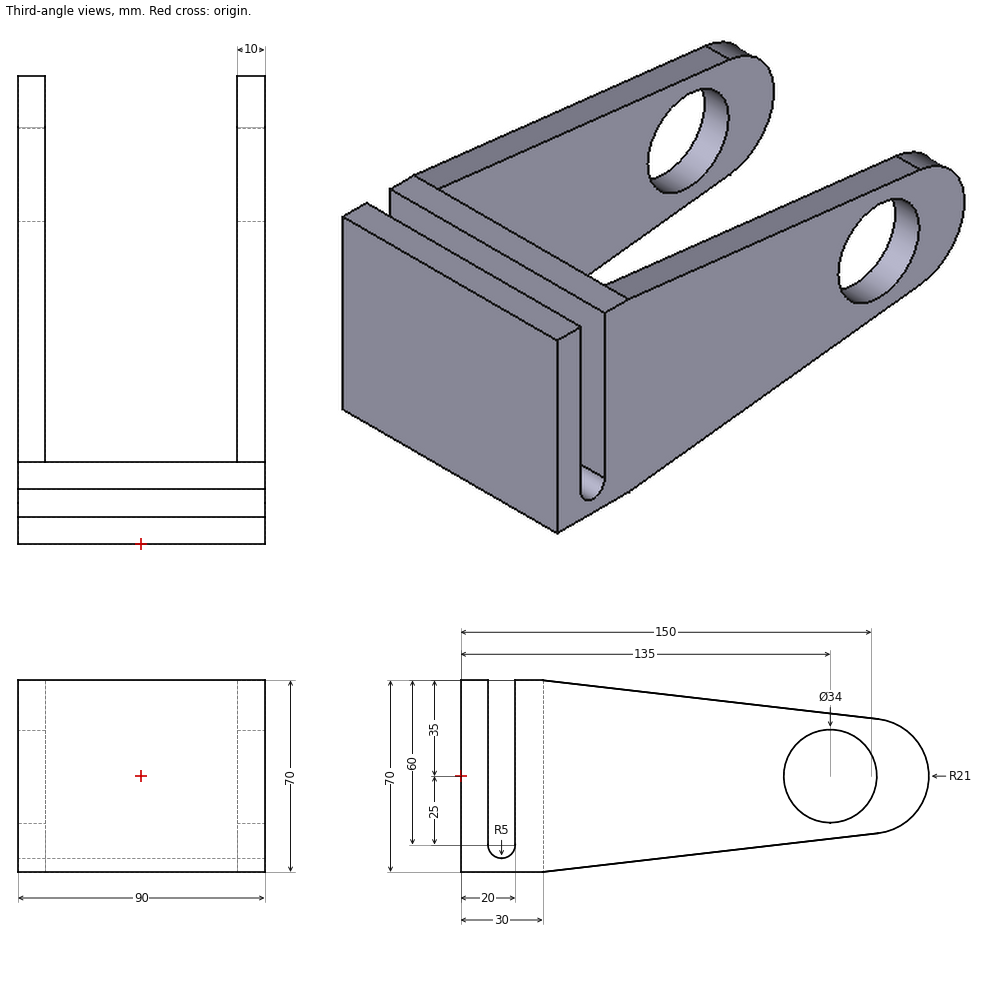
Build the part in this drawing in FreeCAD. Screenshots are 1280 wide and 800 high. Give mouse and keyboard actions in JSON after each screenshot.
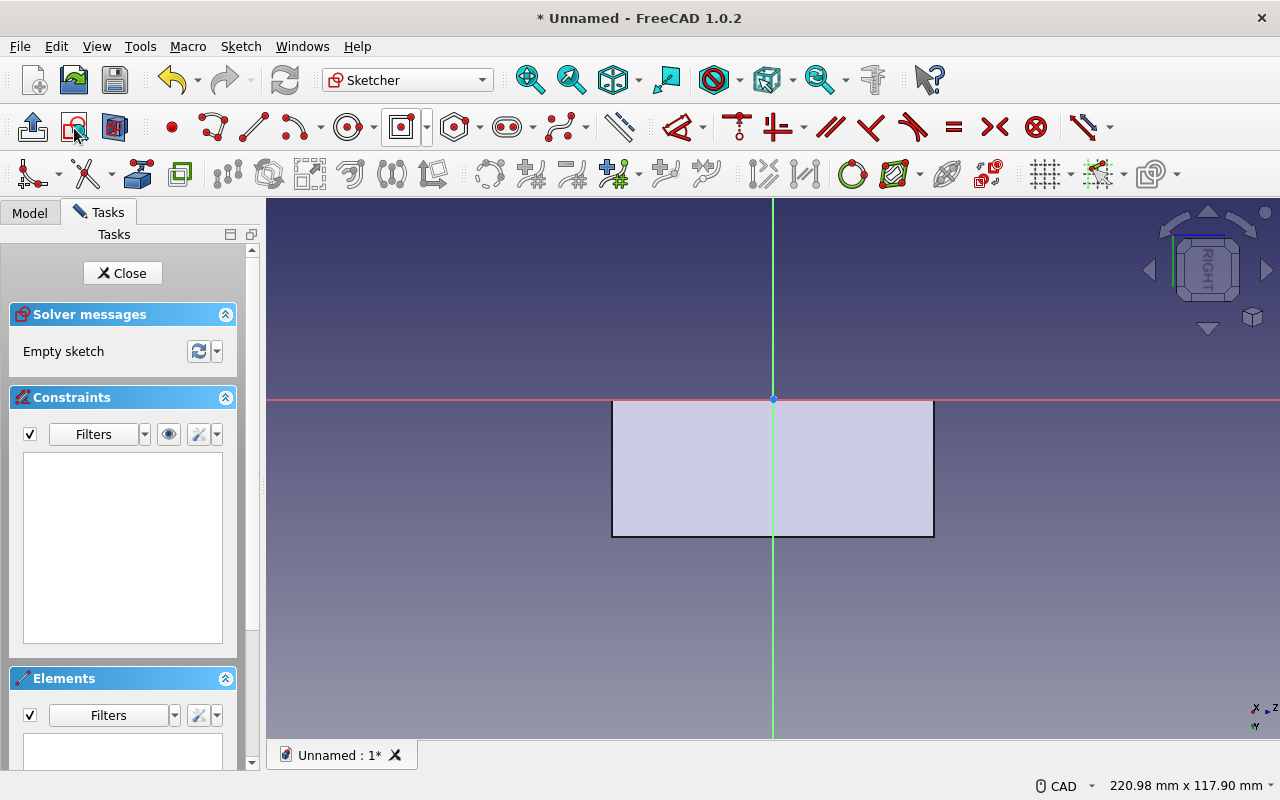
{"action": "scroll", "coordinate": [649, 226], "scroll_direction": "down", "scroll_amount": 4}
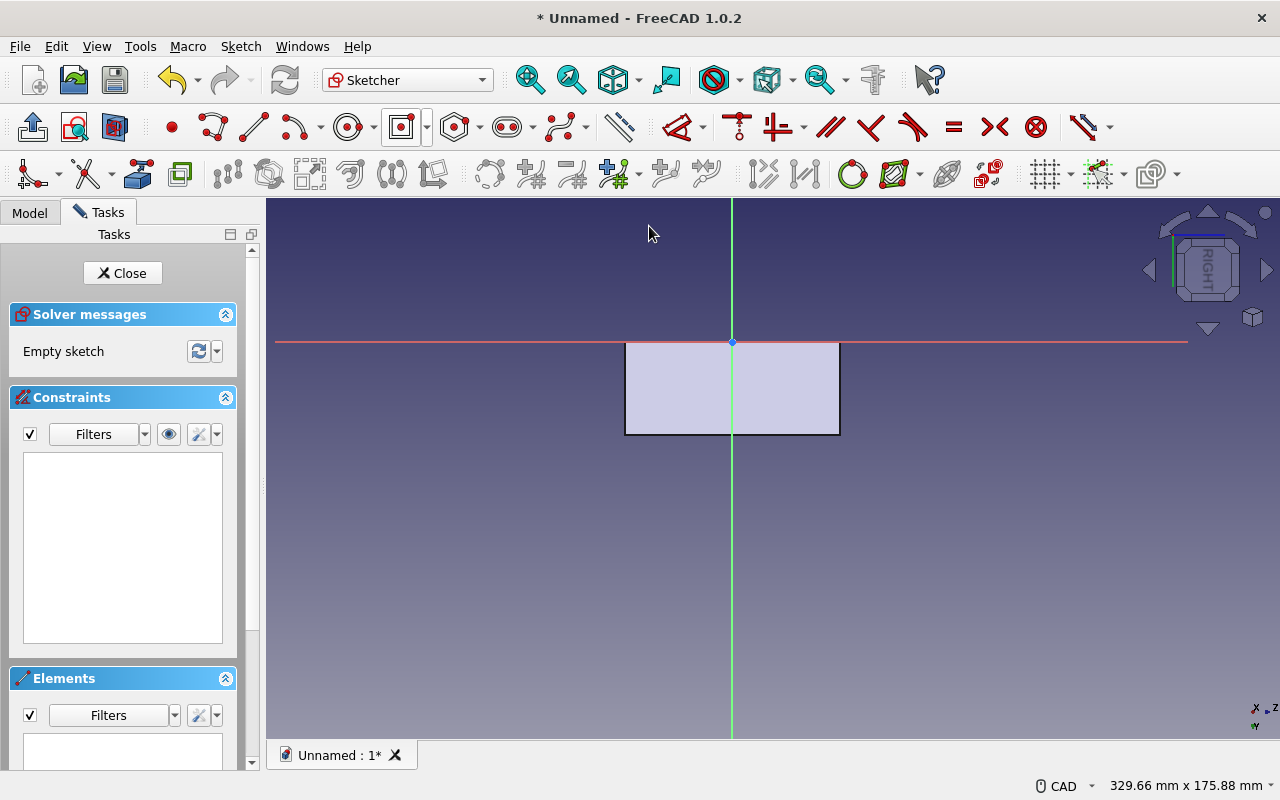
{"action": "left_click", "coordinate": [213, 128]}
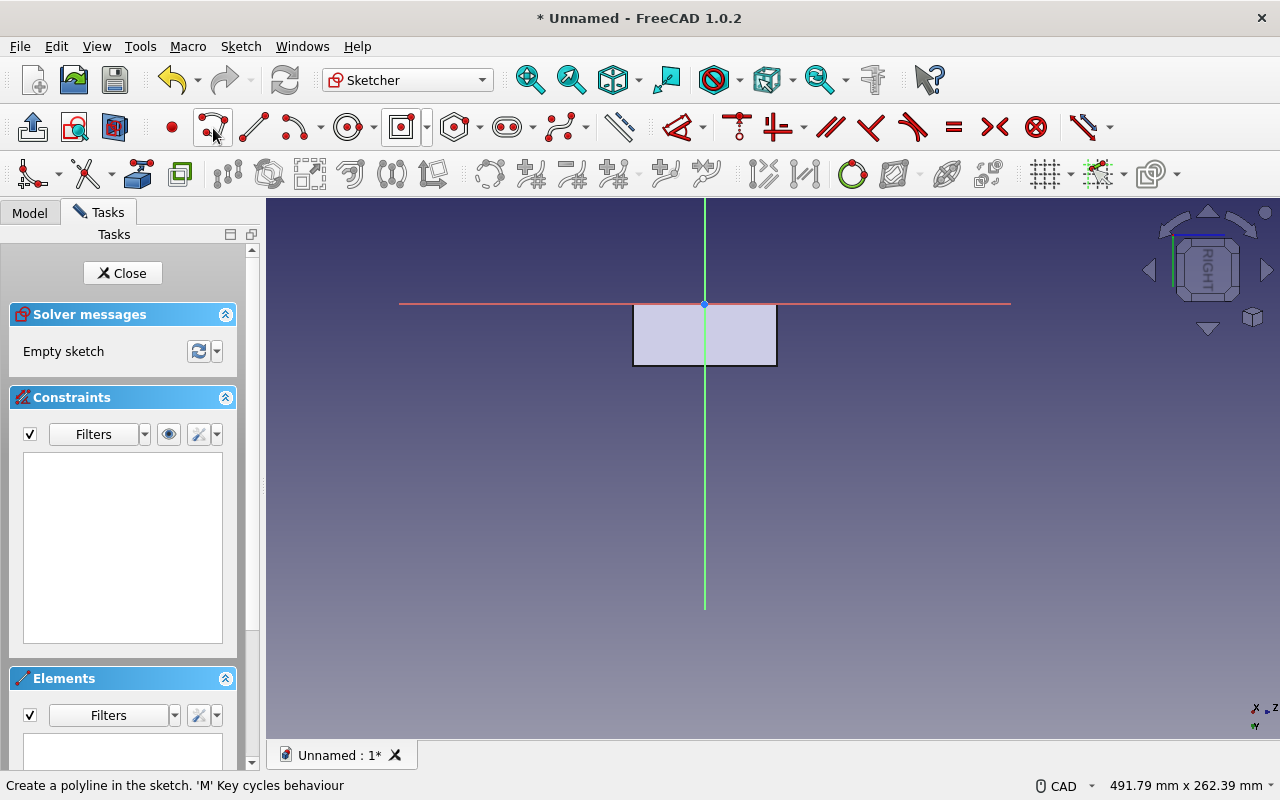
{"action": "left_click", "coordinate": [748, 618]}
{"action": "left_click", "coordinate": [777, 366]}
{"action": "left_click", "coordinate": [633, 366]}
{"action": "left_click", "coordinate": [662, 618]}
{"action": "right_click", "coordinate": [662, 618]}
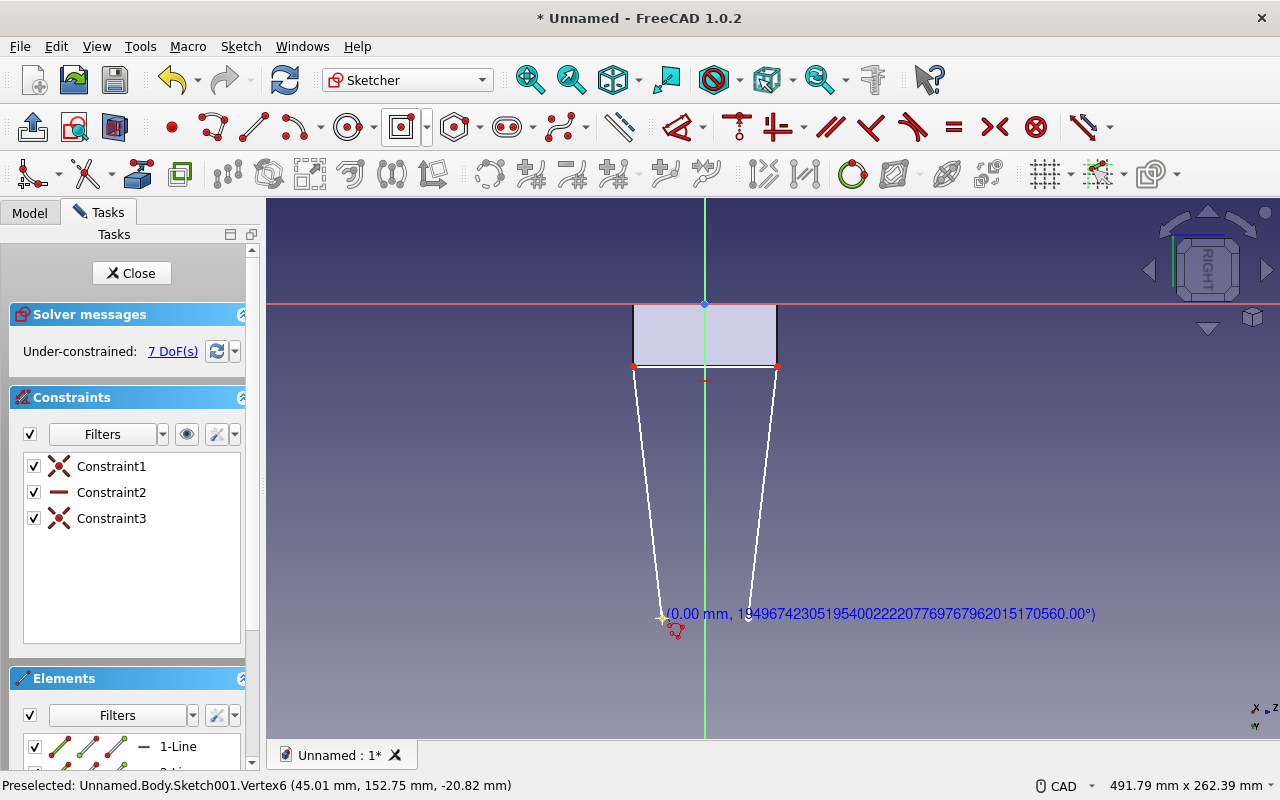
{"action": "left_click", "coordinate": [320, 128]}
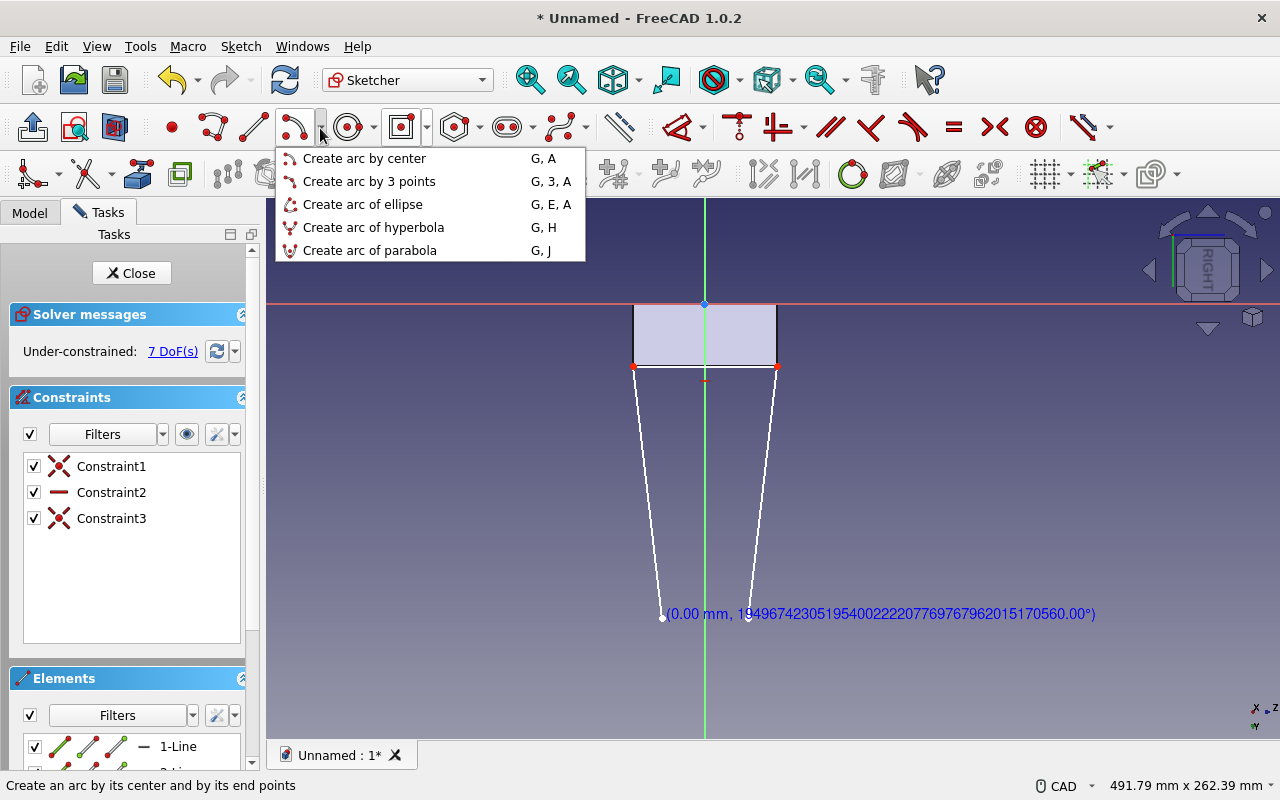
{"action": "left_click", "coordinate": [430, 182]}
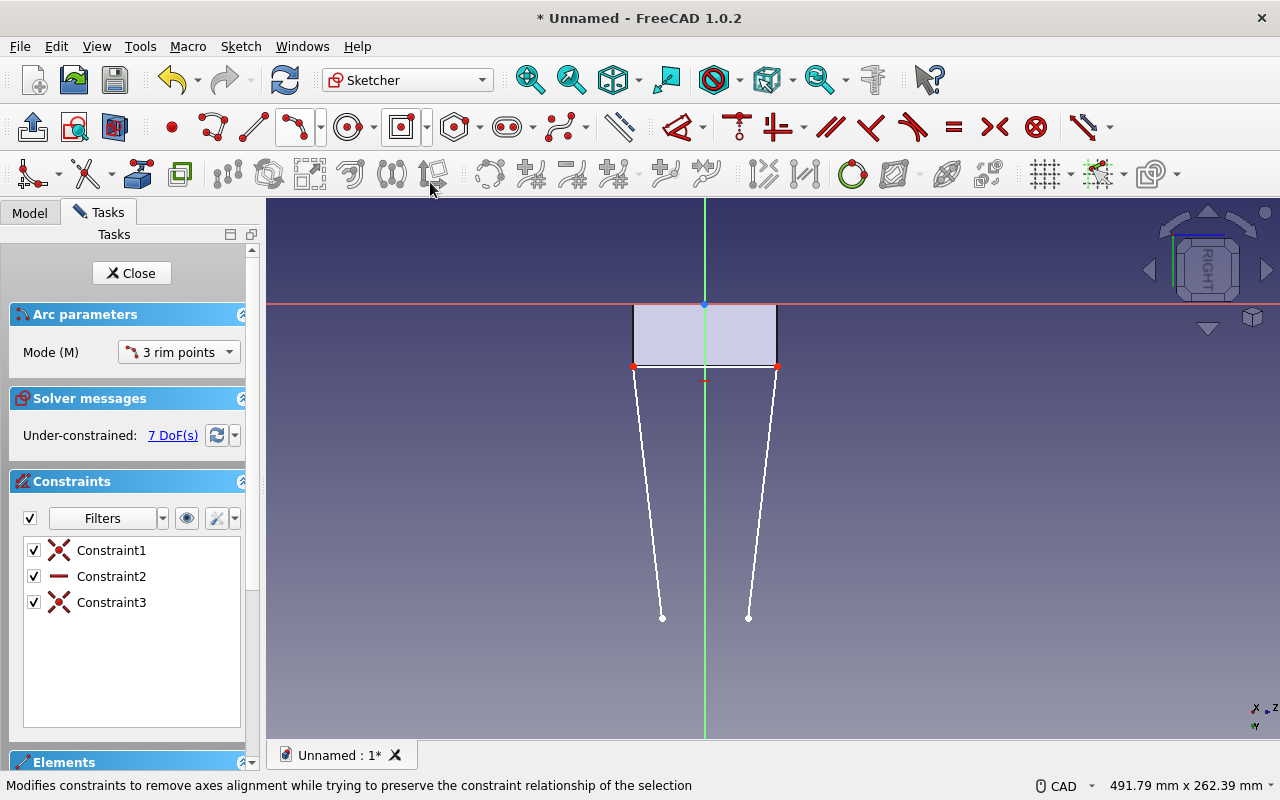
{"action": "left_click", "coordinate": [662, 619]}
{"action": "left_click", "coordinate": [748, 619]}
{"action": "left_click", "coordinate": [681, 650]}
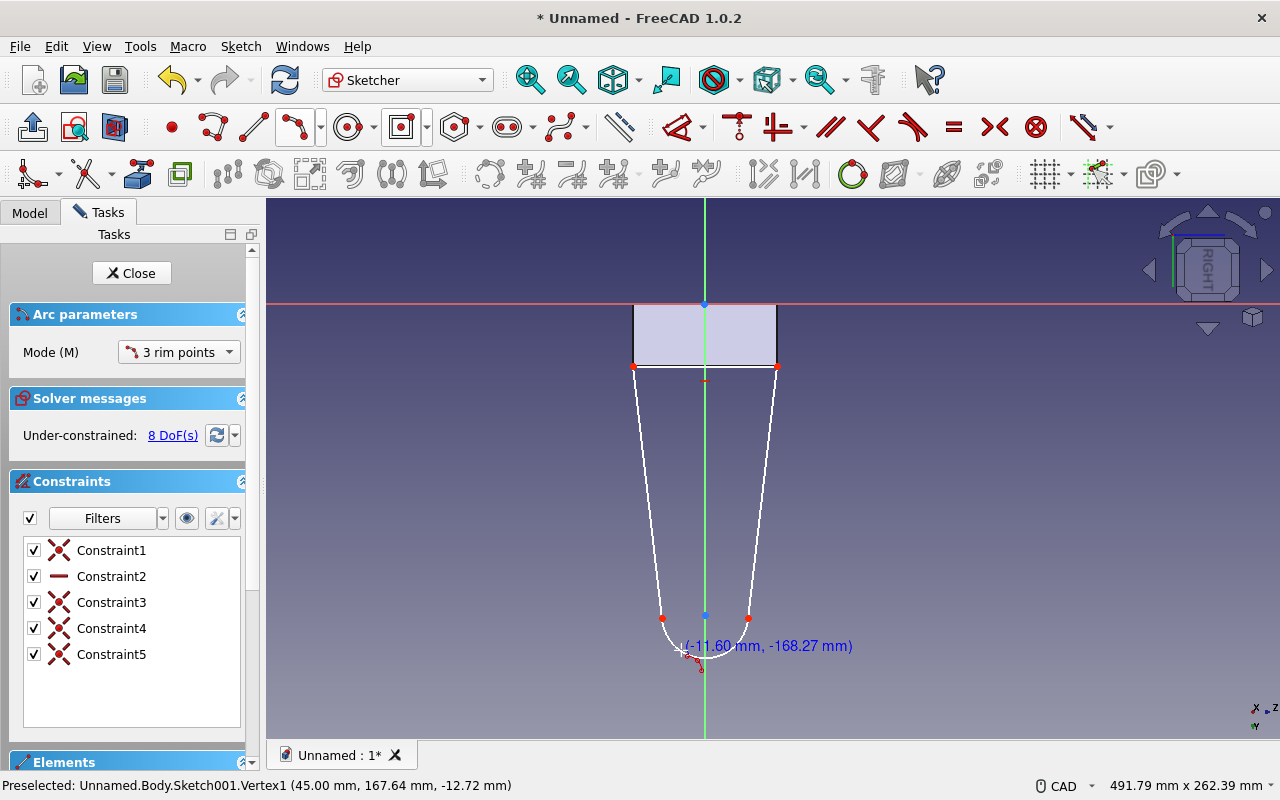
{"action": "left_click", "coordinate": [348, 128]}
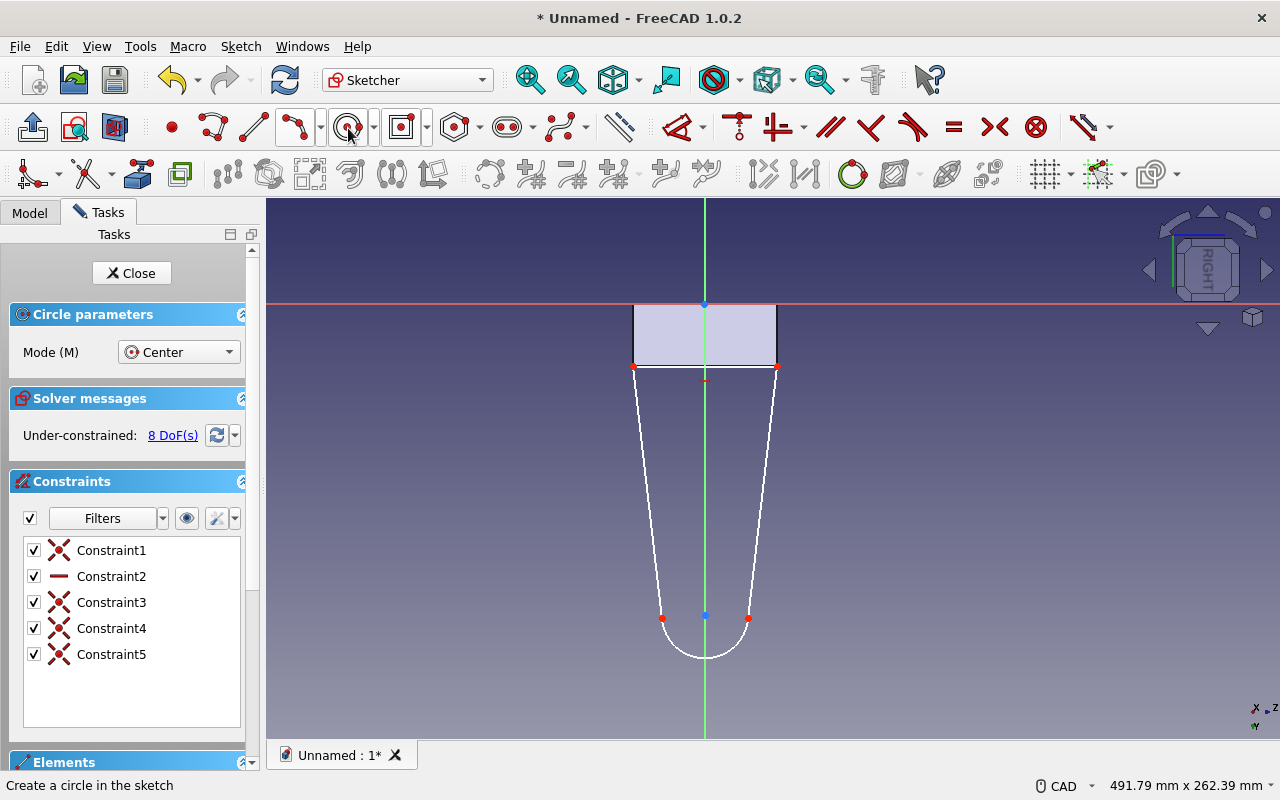
{"action": "left_click", "coordinate": [705, 582]}
{"action": "left_click", "coordinate": [730, 558]}
{"action": "key", "text": "Escape"}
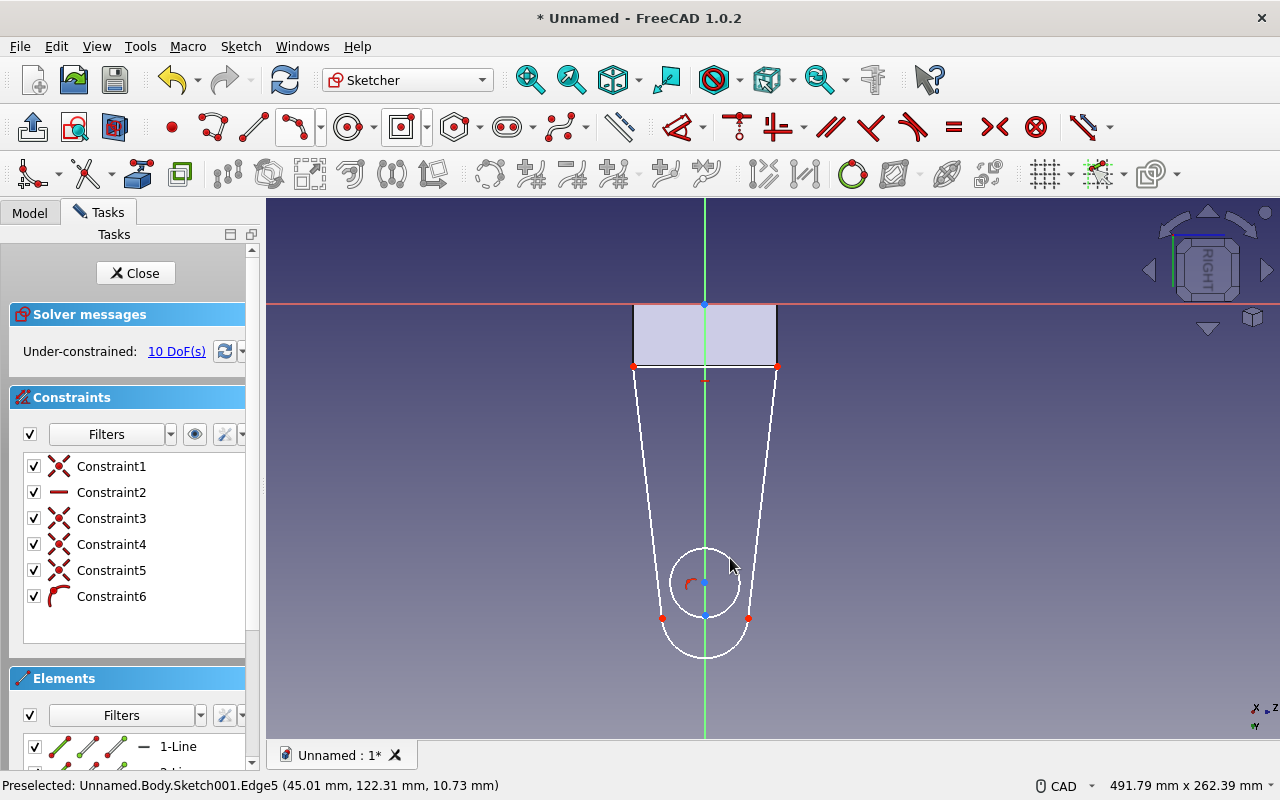
{"action": "left_click", "coordinate": [757, 543]}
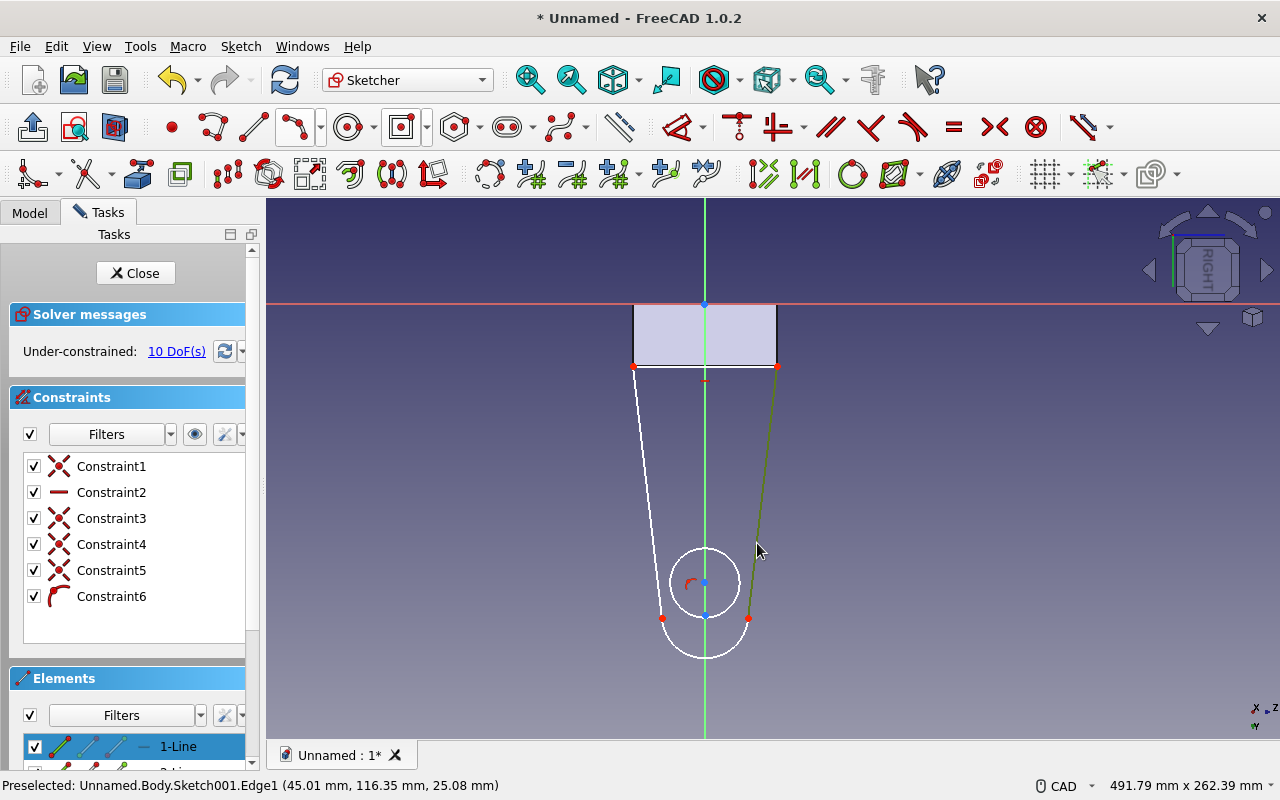
{"action": "left_click", "coordinate": [681, 651]}